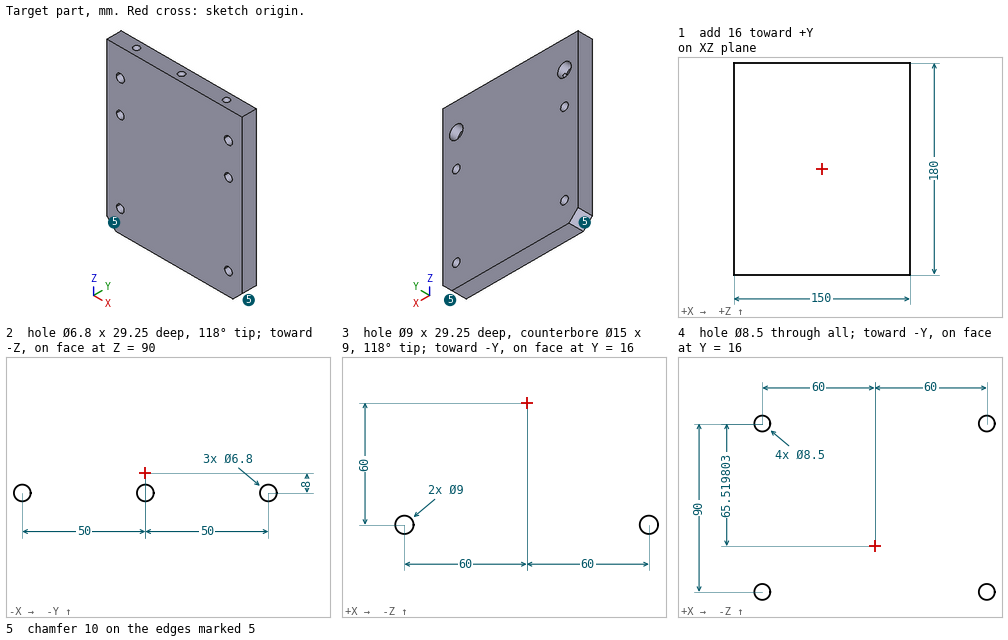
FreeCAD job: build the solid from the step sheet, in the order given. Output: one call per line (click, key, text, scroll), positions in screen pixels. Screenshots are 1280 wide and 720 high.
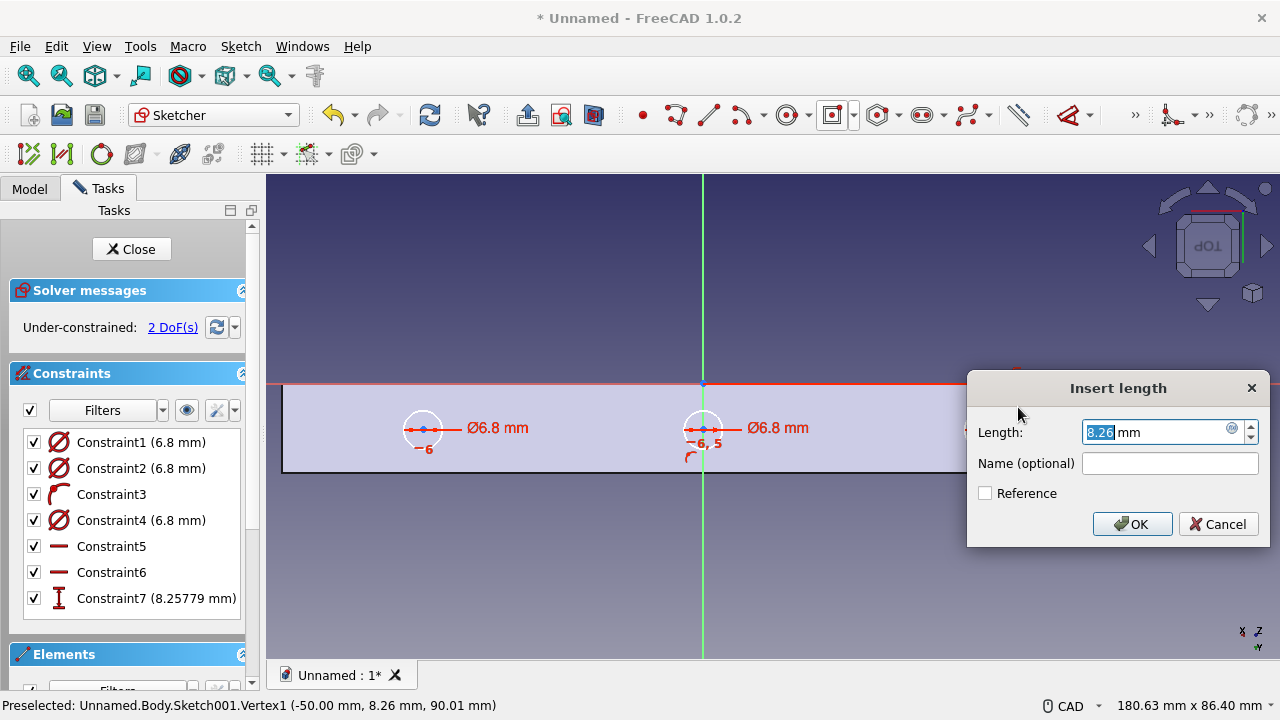
text(8)
key(Return)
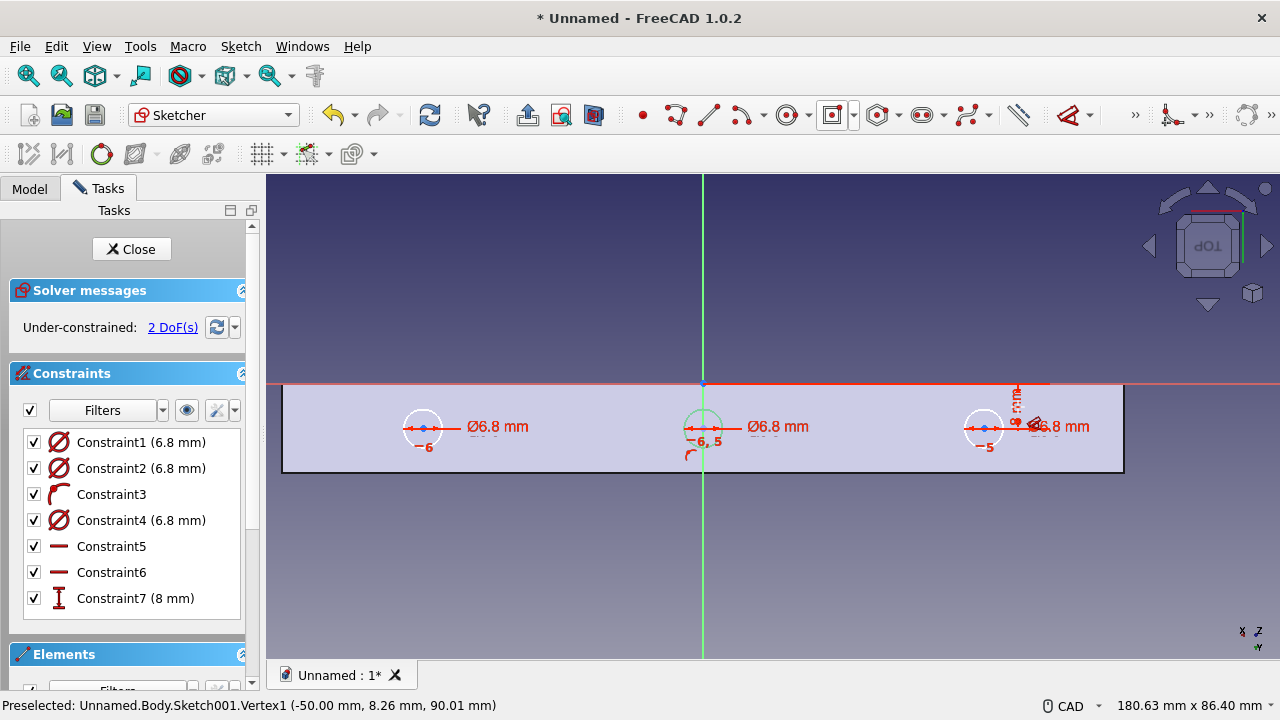
click(984, 429)
click(844, 350)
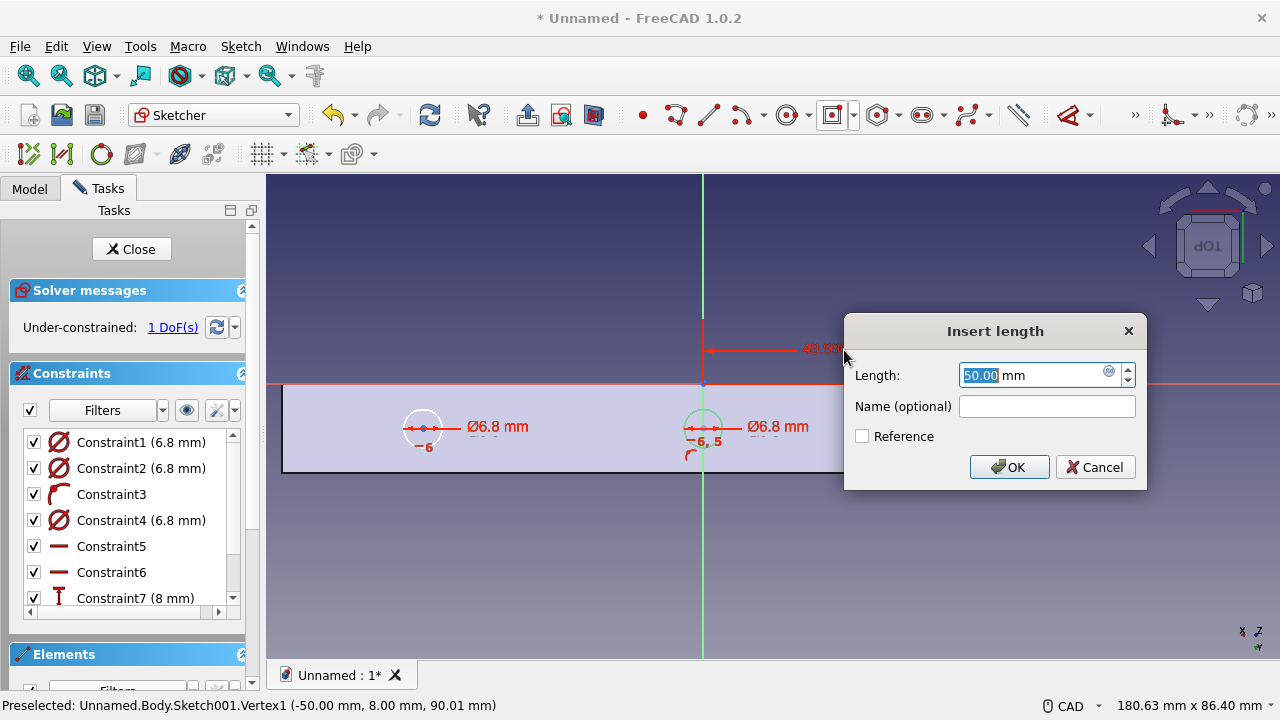
text(50)
key(Return)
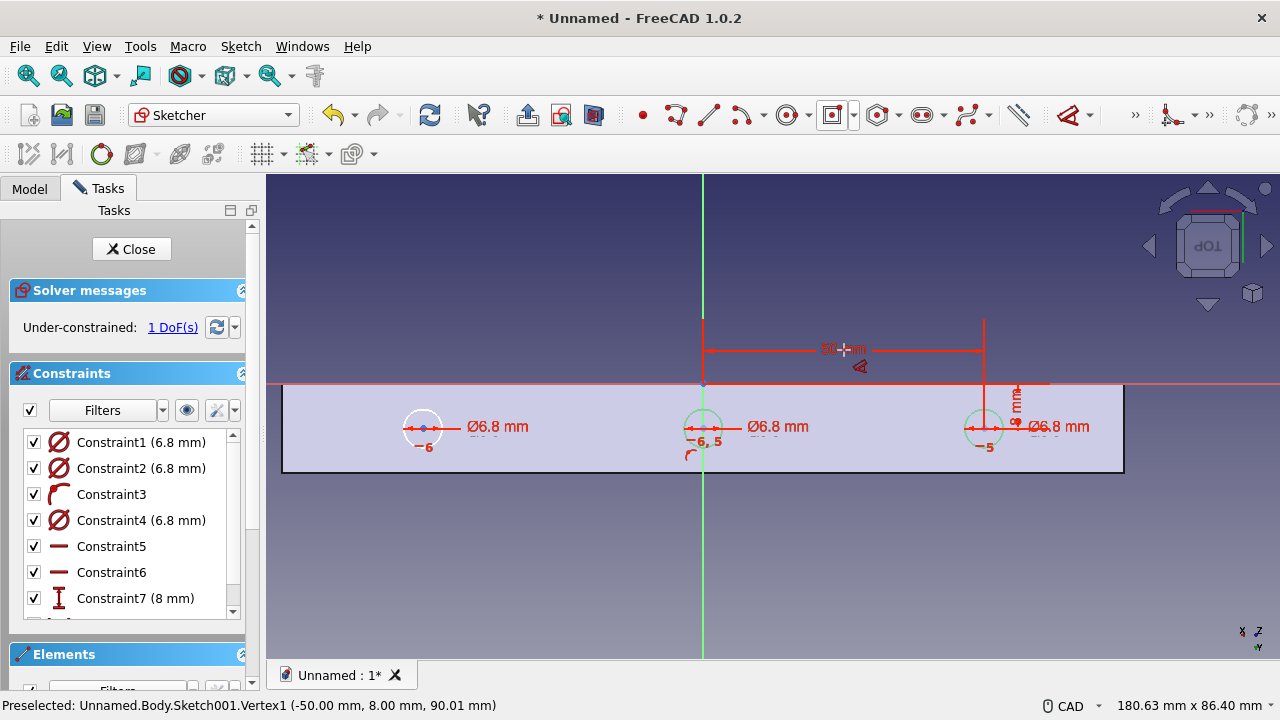
click(423, 429)
click(563, 350)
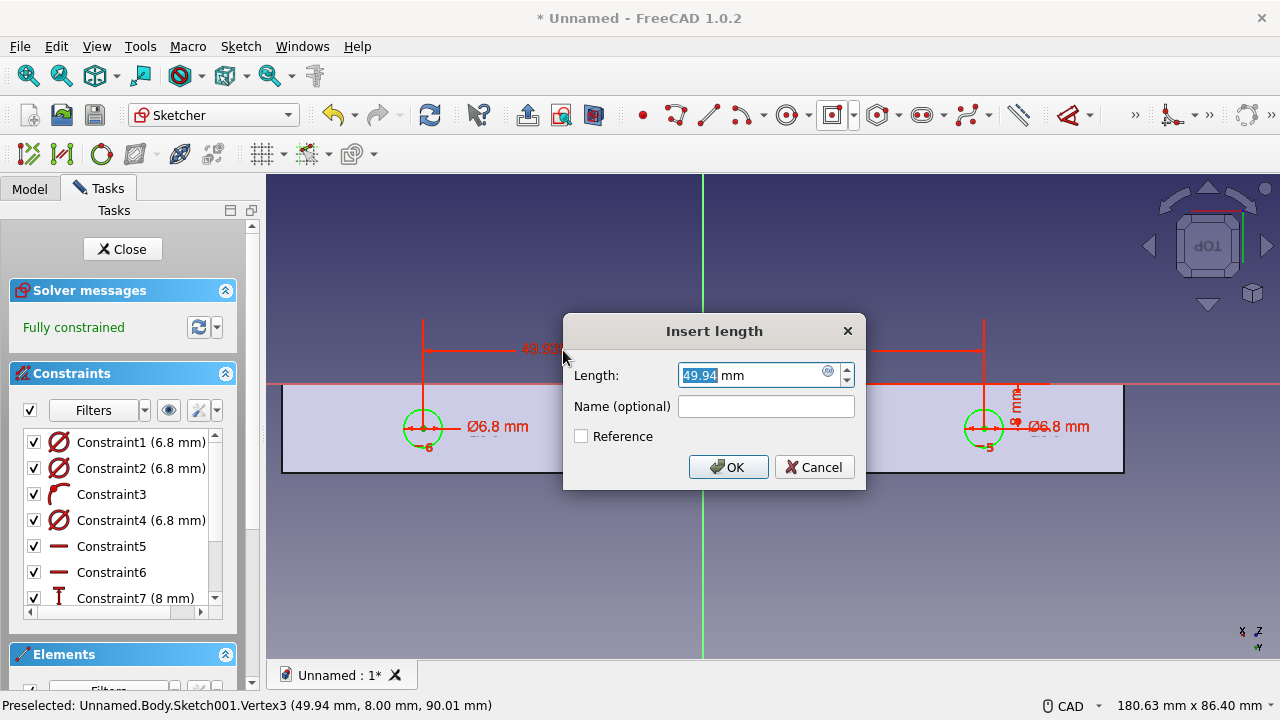
text(50)
key(Return)
key(Escape)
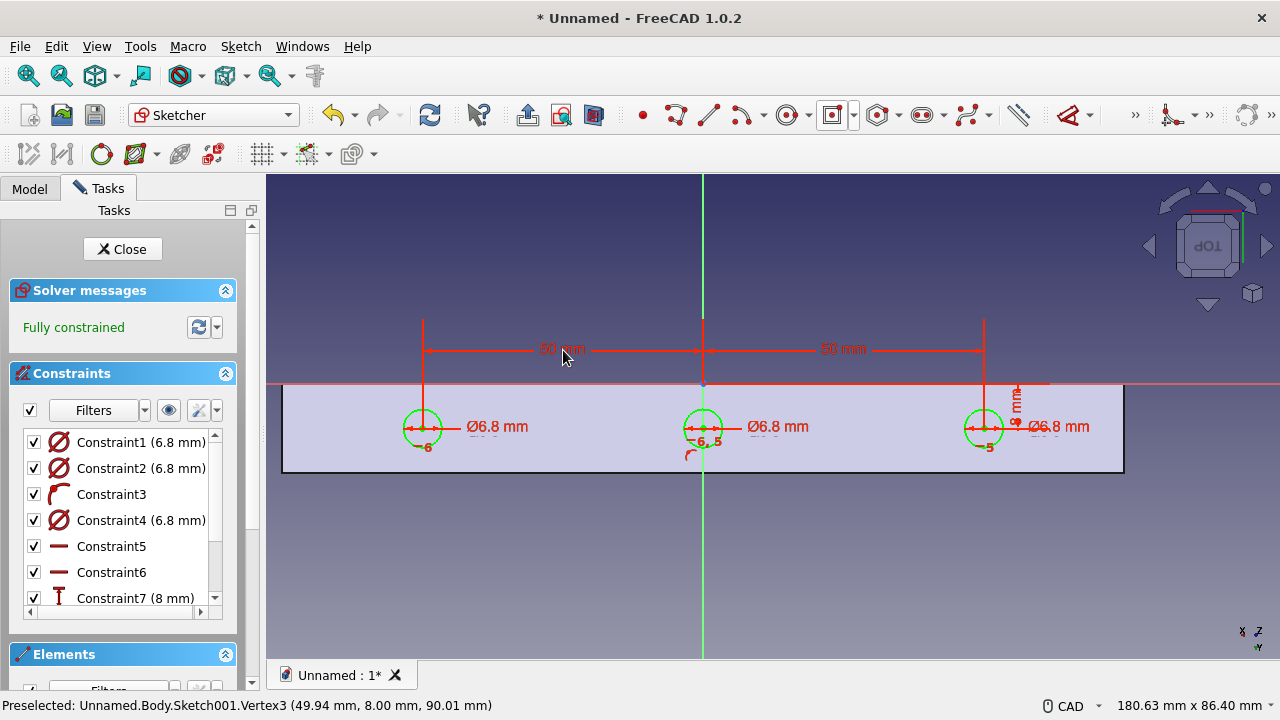
click(123, 249)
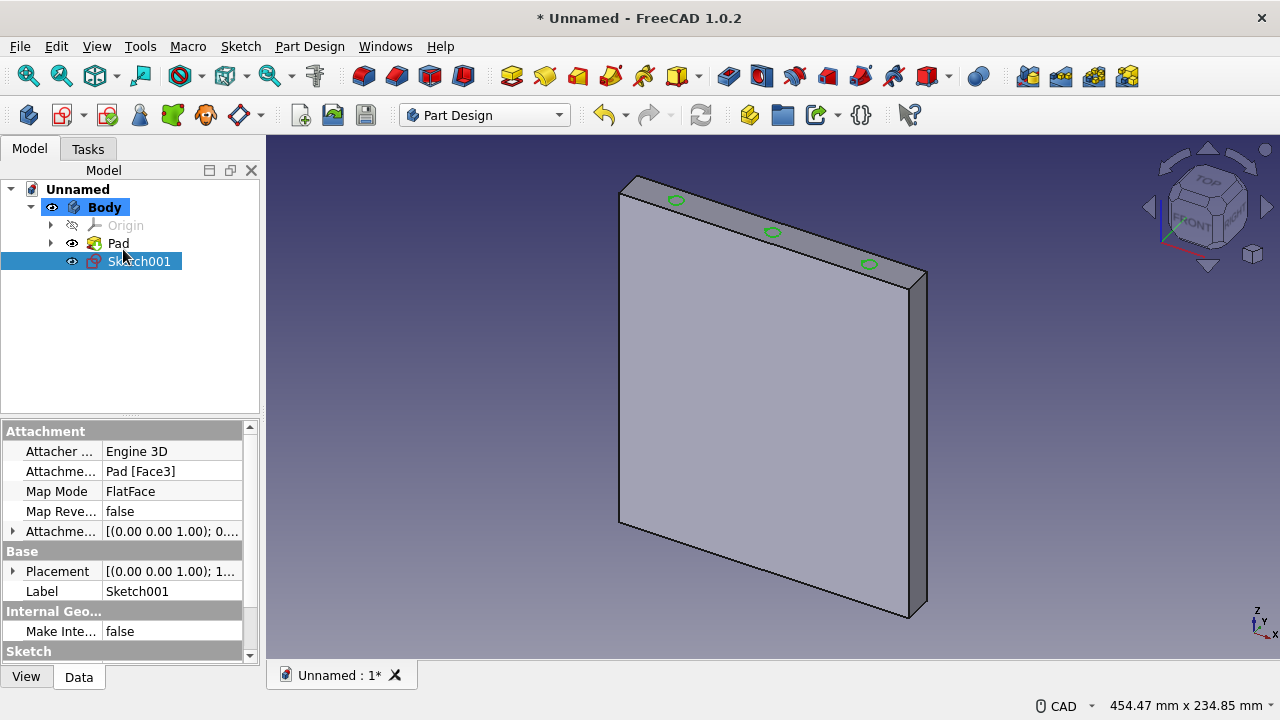
click(762, 76)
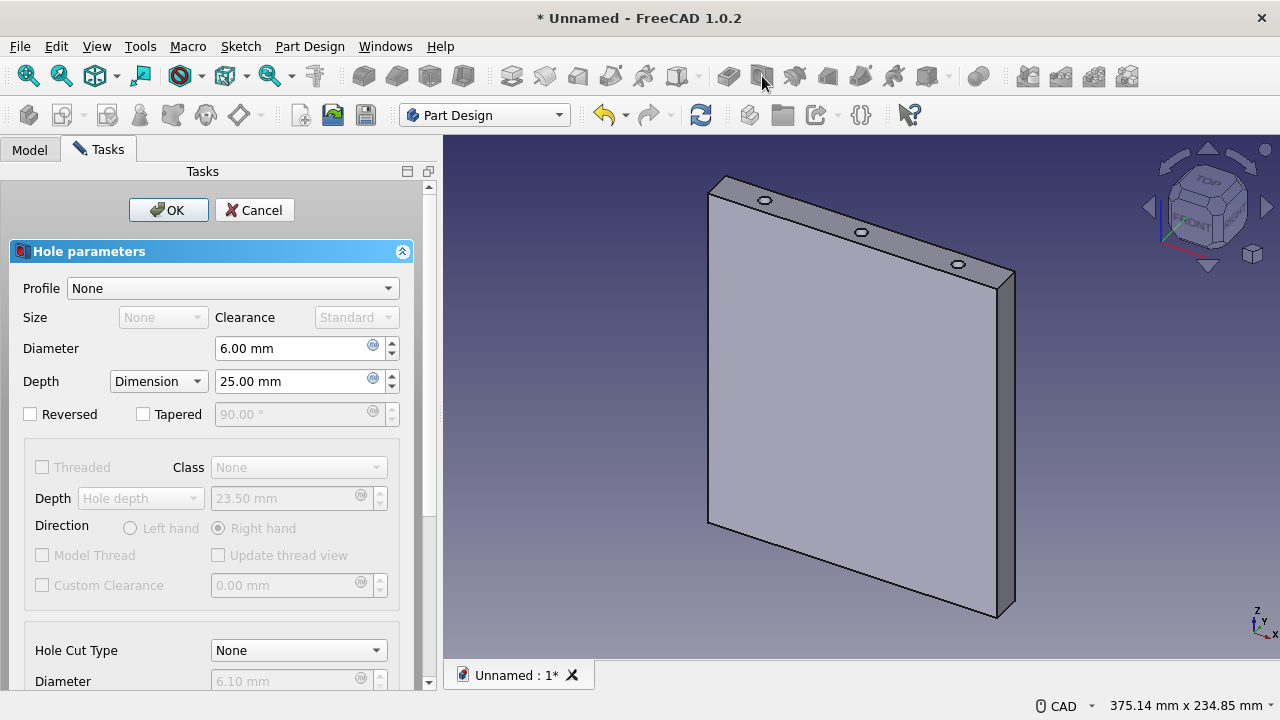
triple_click(300, 348)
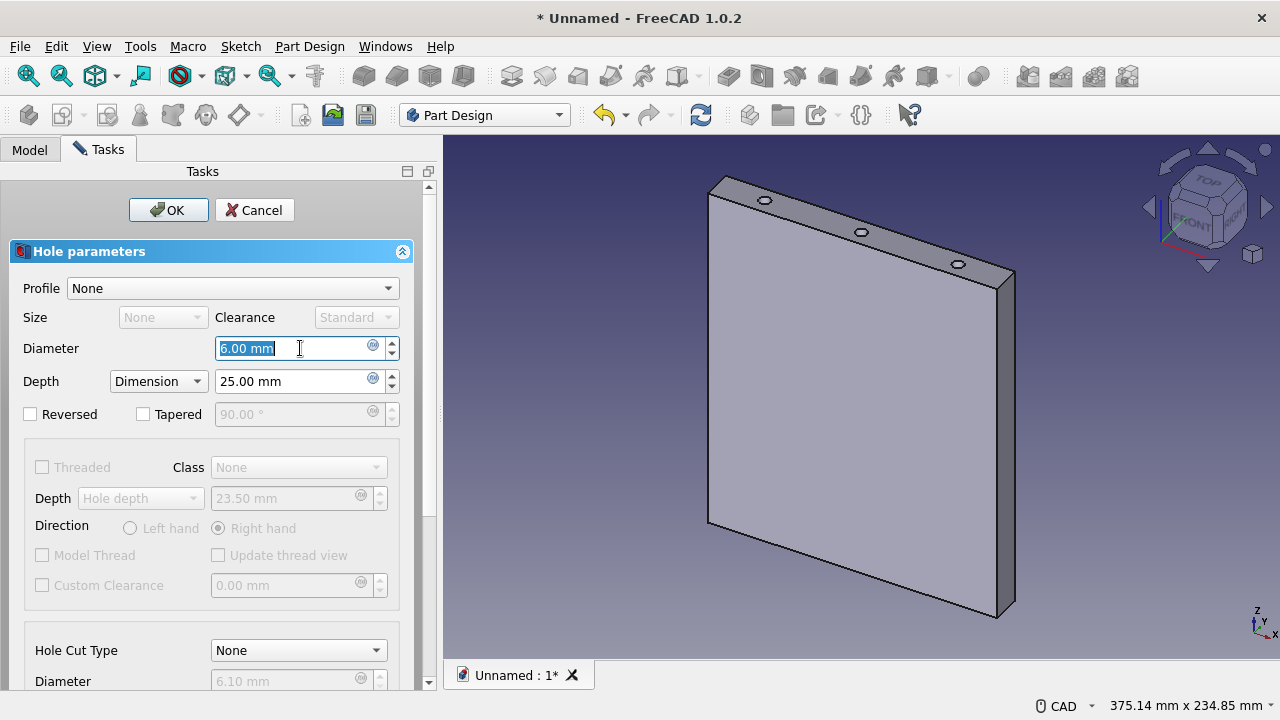
text(6.8)
key(Tab)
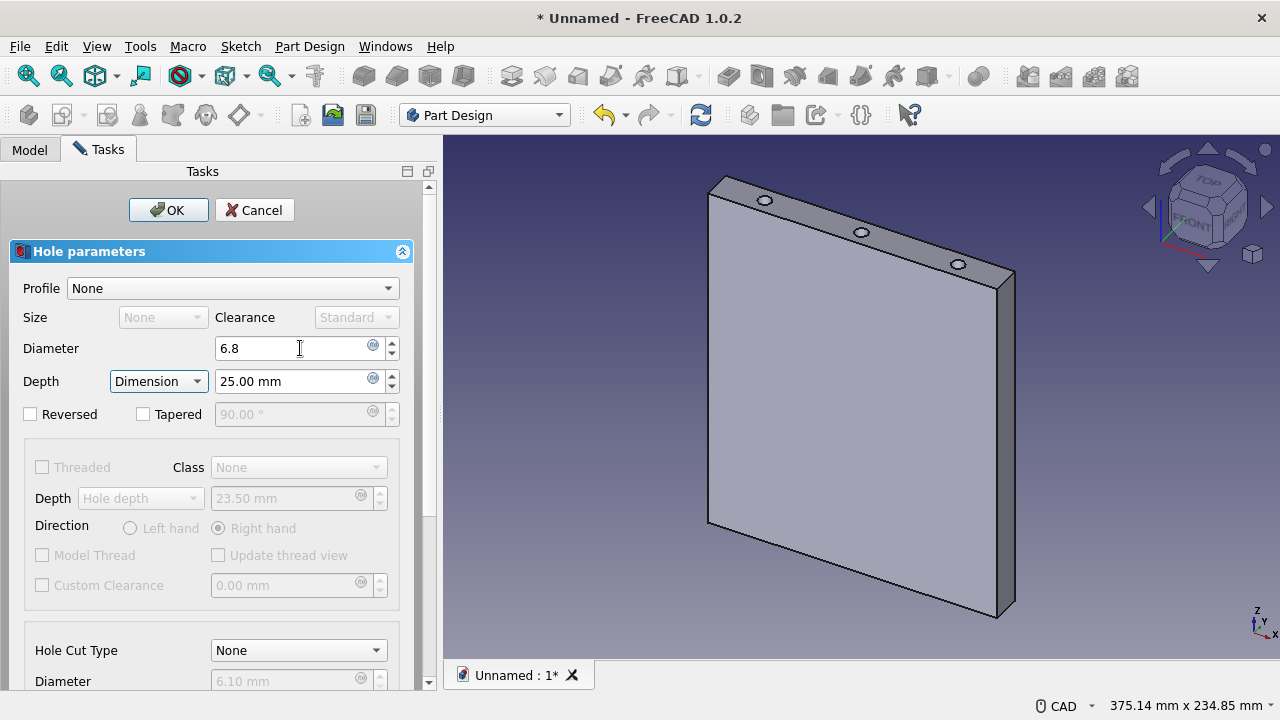
triple_click(300, 382)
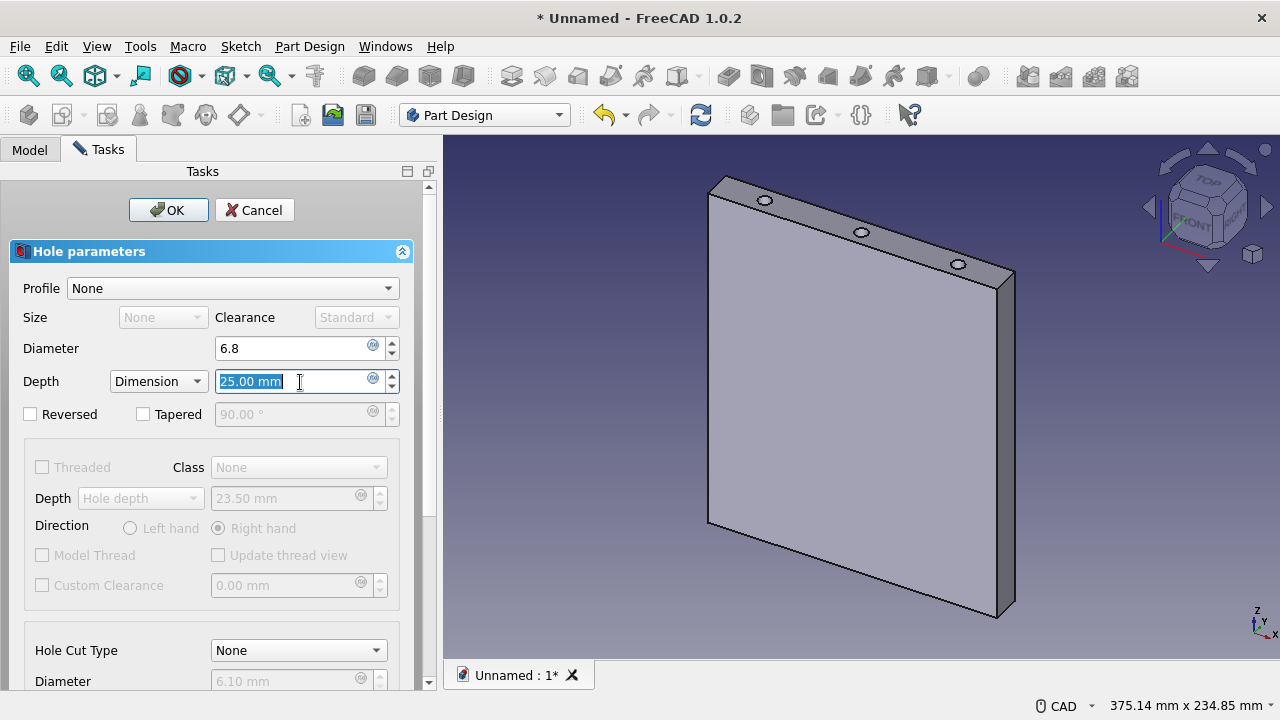
text(29.25)
key(Tab)